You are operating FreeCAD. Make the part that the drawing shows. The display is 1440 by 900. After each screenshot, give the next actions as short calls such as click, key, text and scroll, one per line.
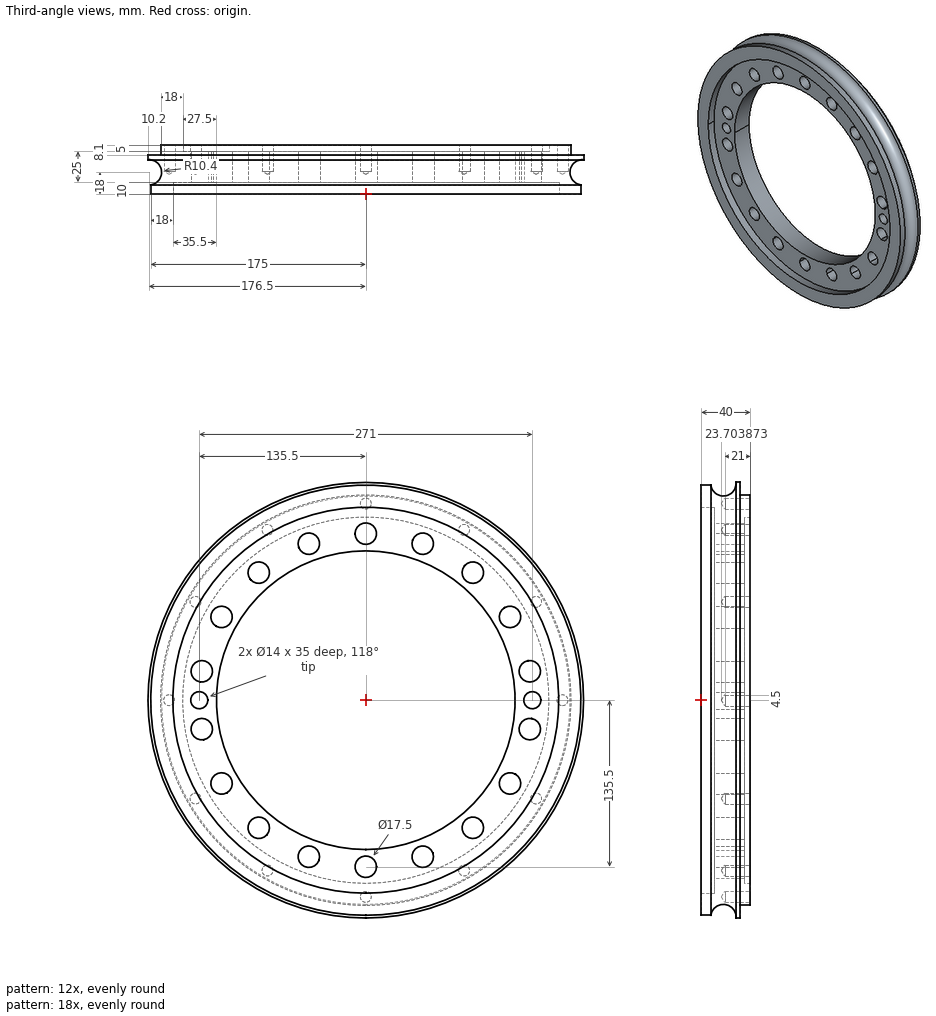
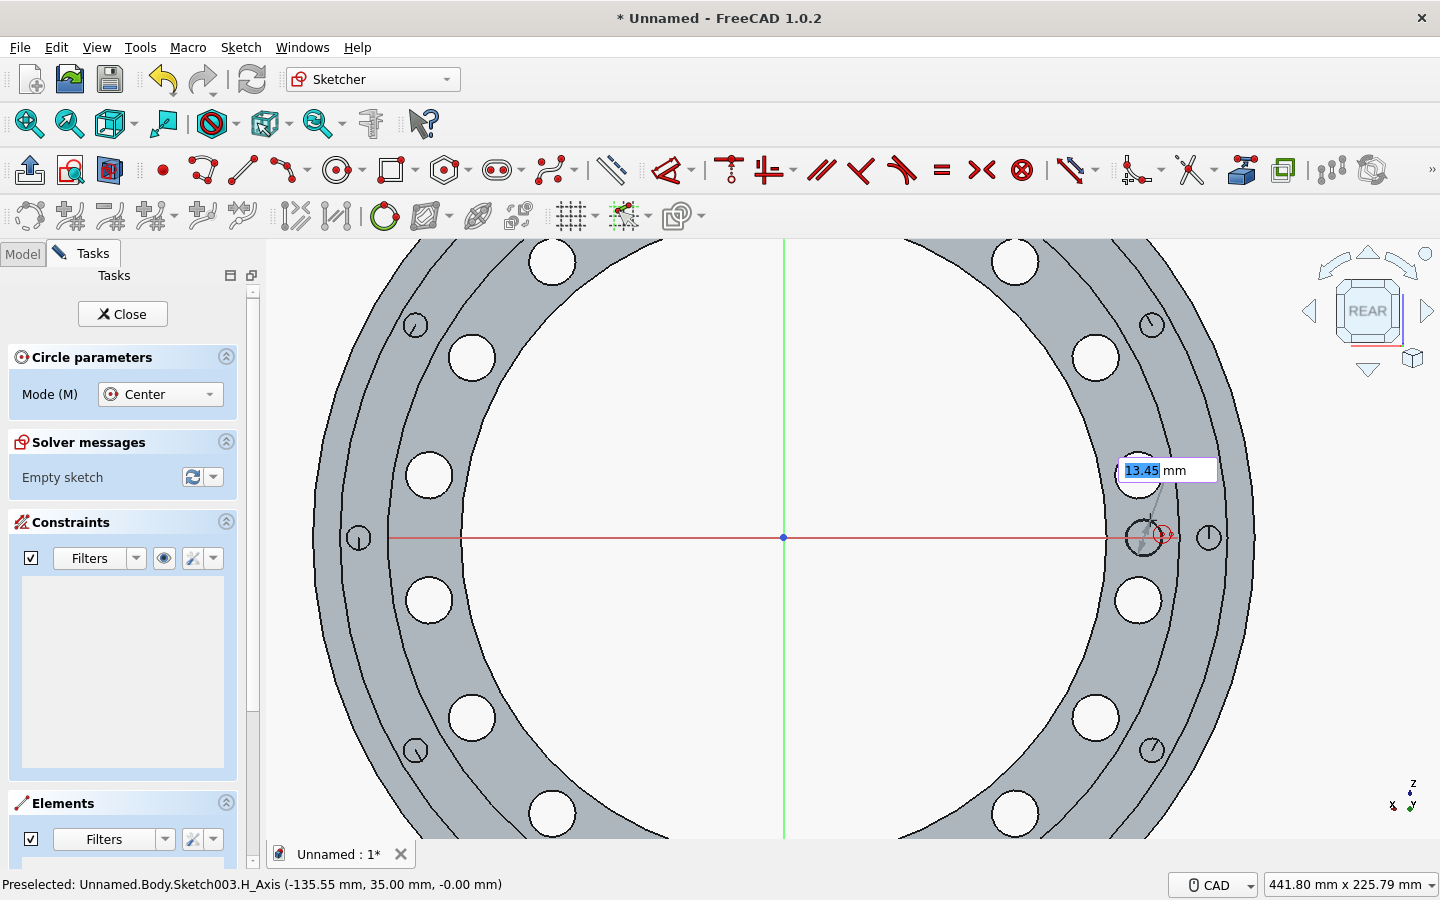
text(14)
key(Return)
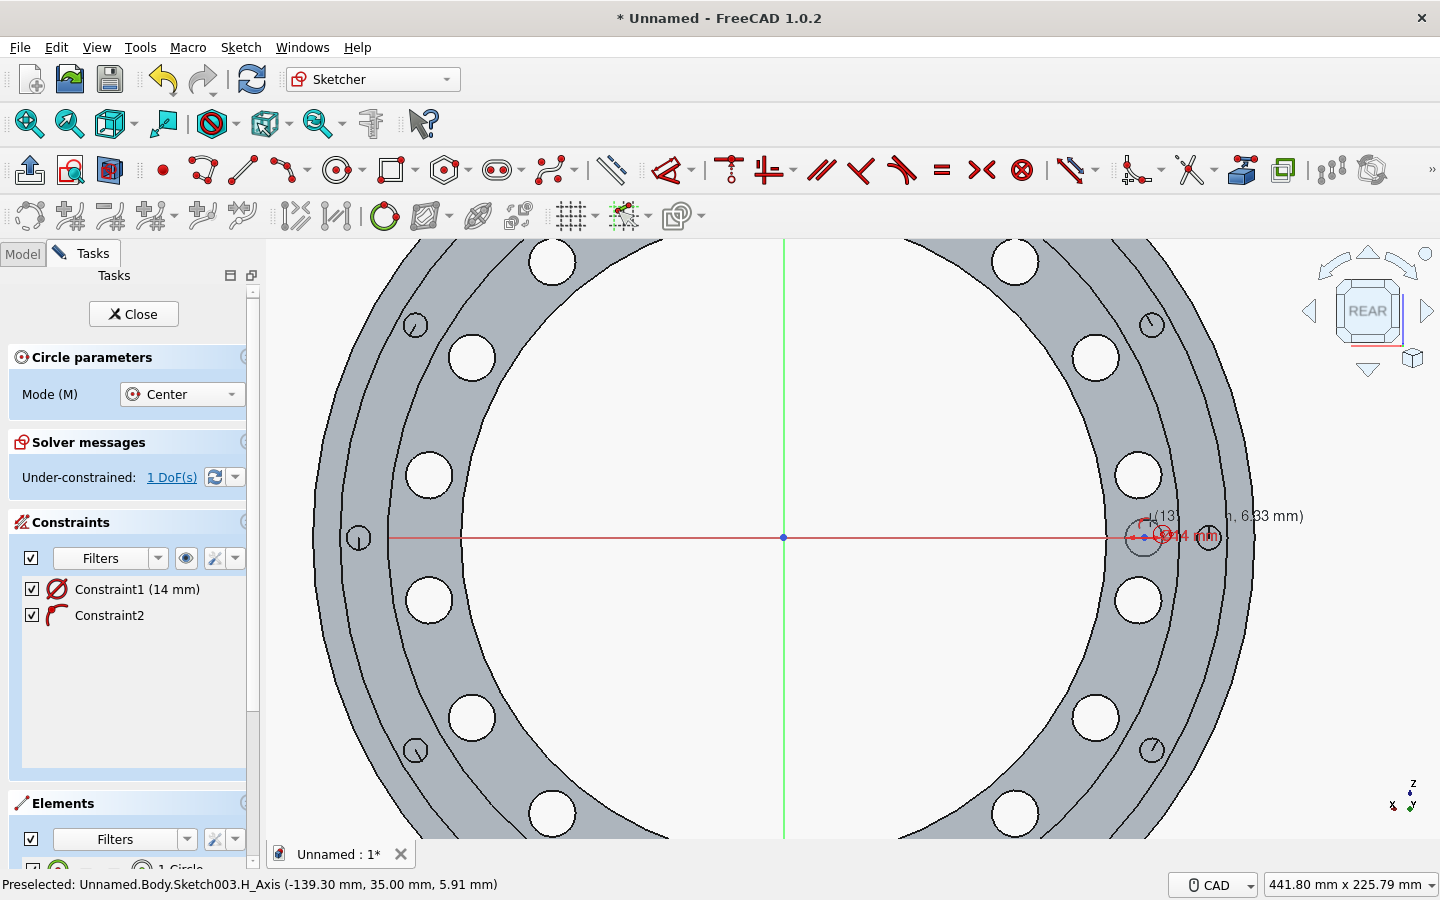
click(424, 538)
move(430, 520)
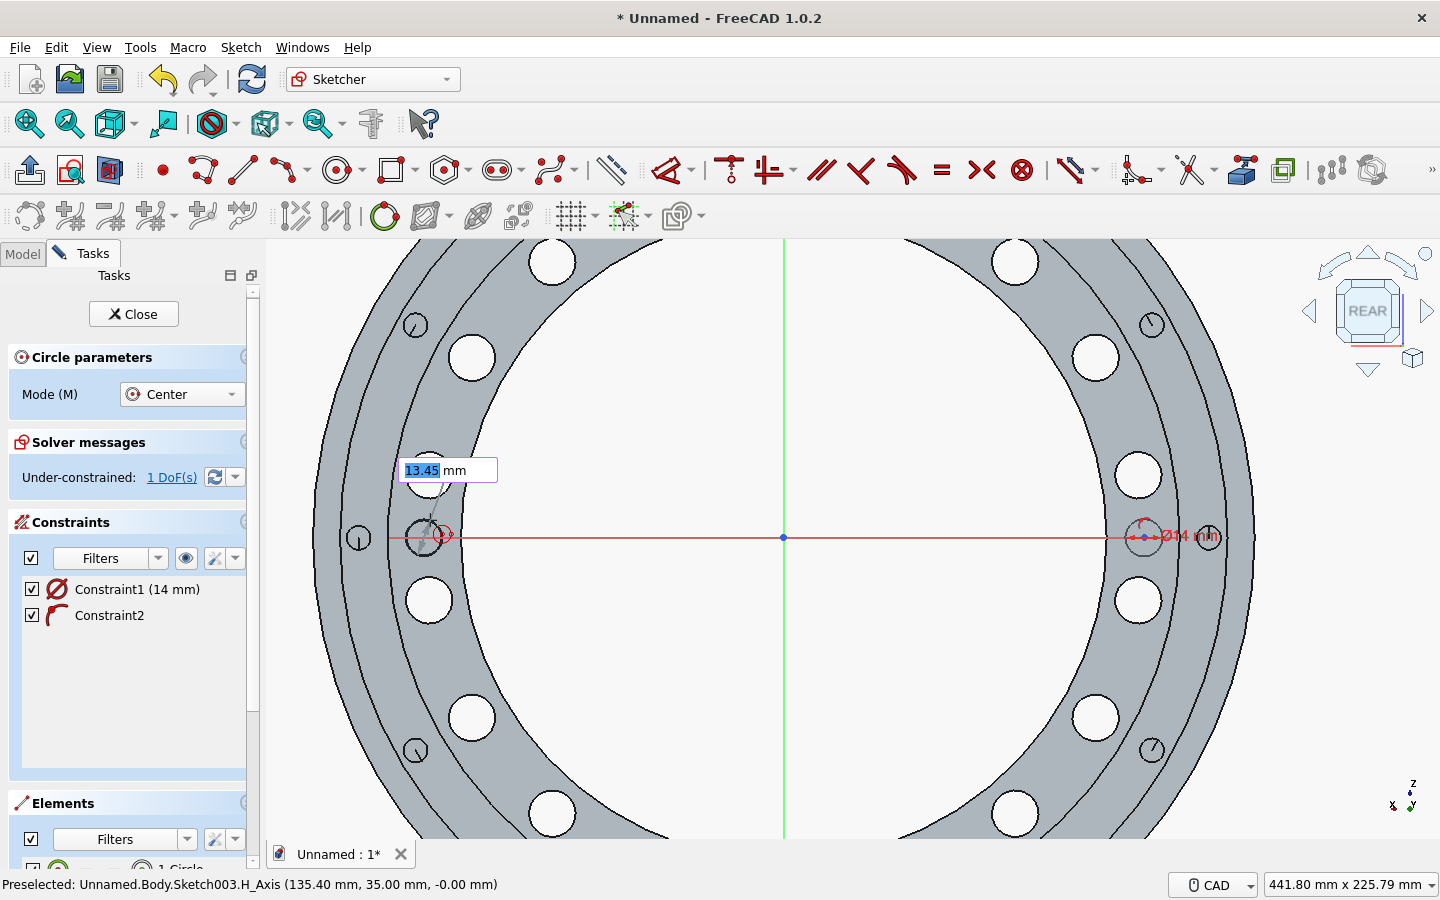
text(14)
key(Return)
key(Escape)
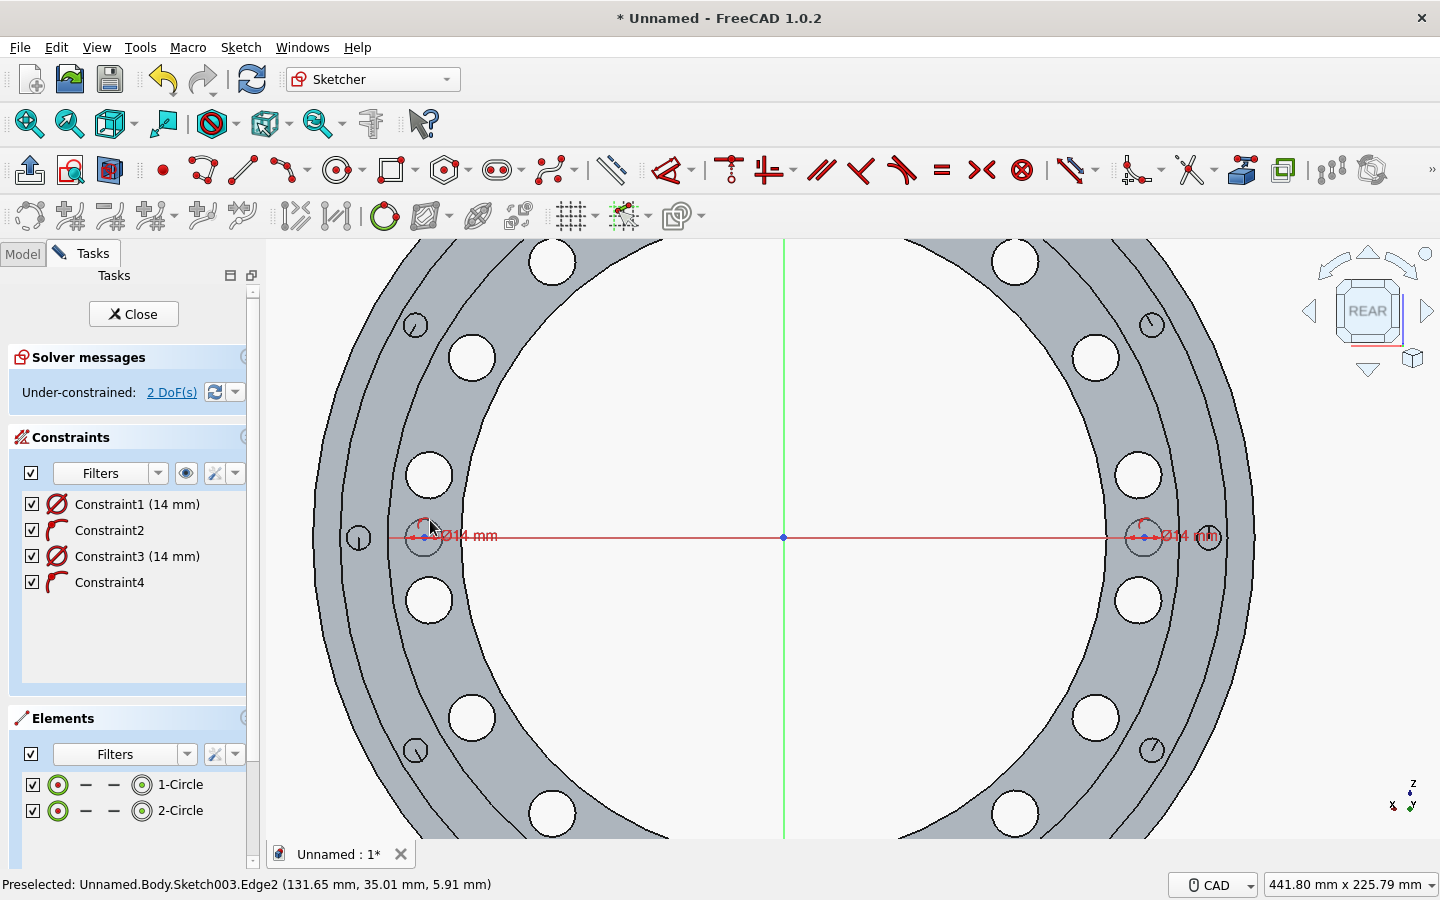
click(666, 170)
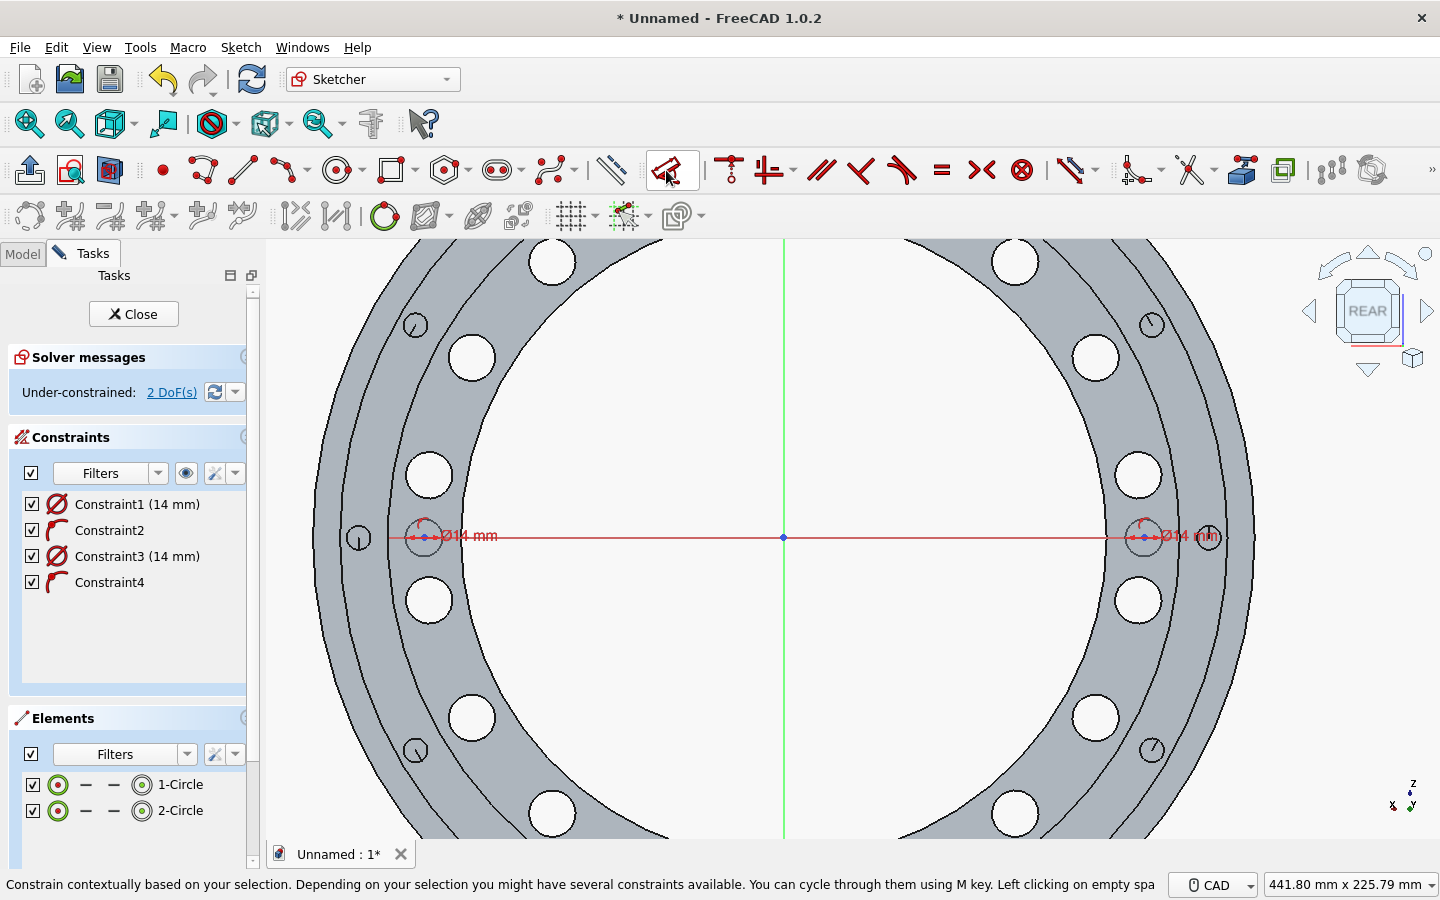
click(1144, 538)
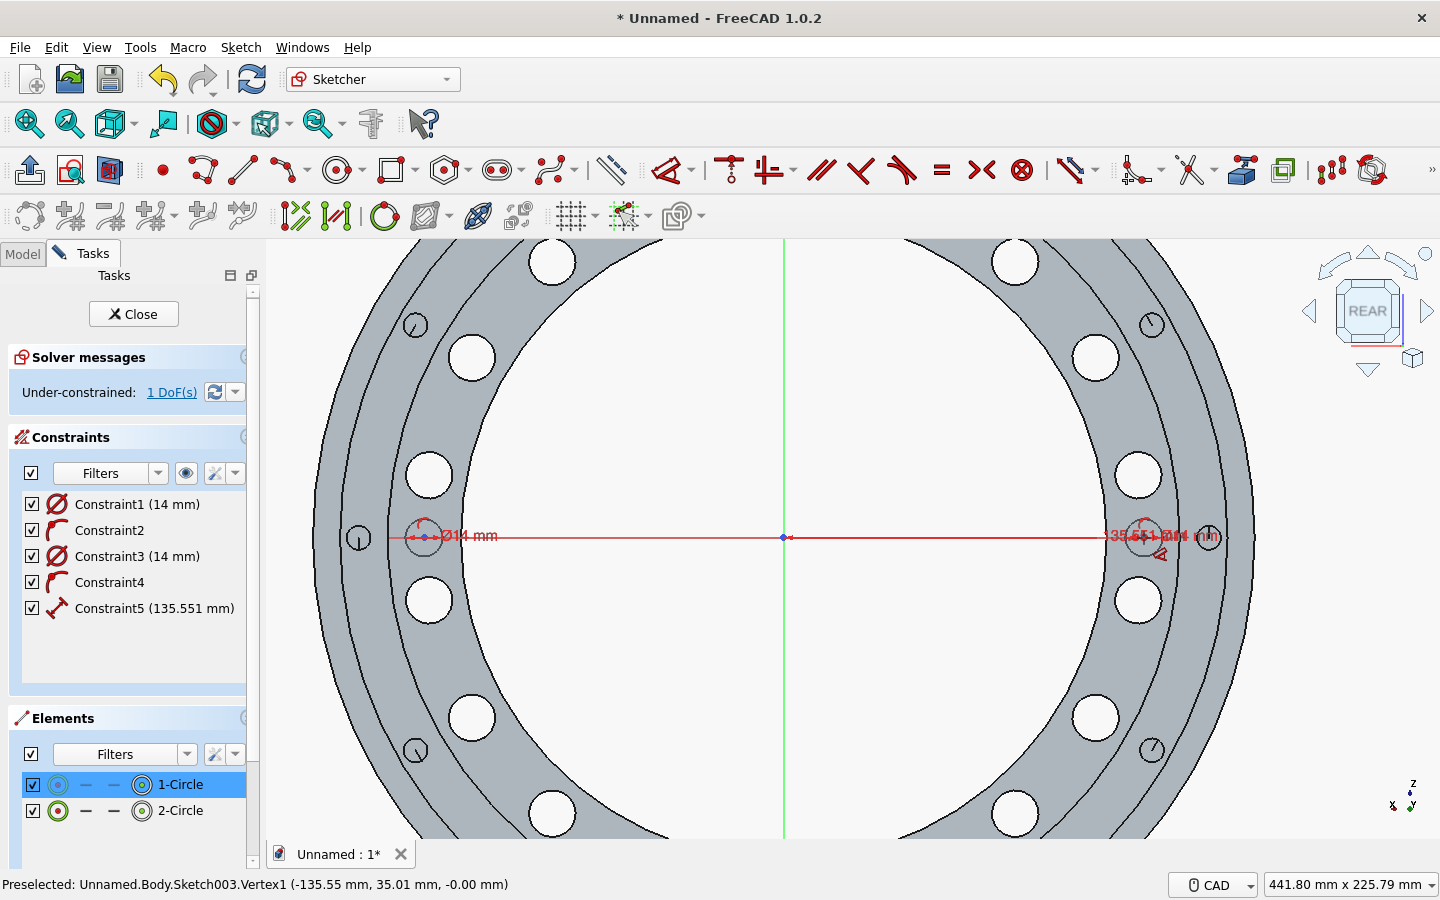
click(424, 538)
click(618, 572)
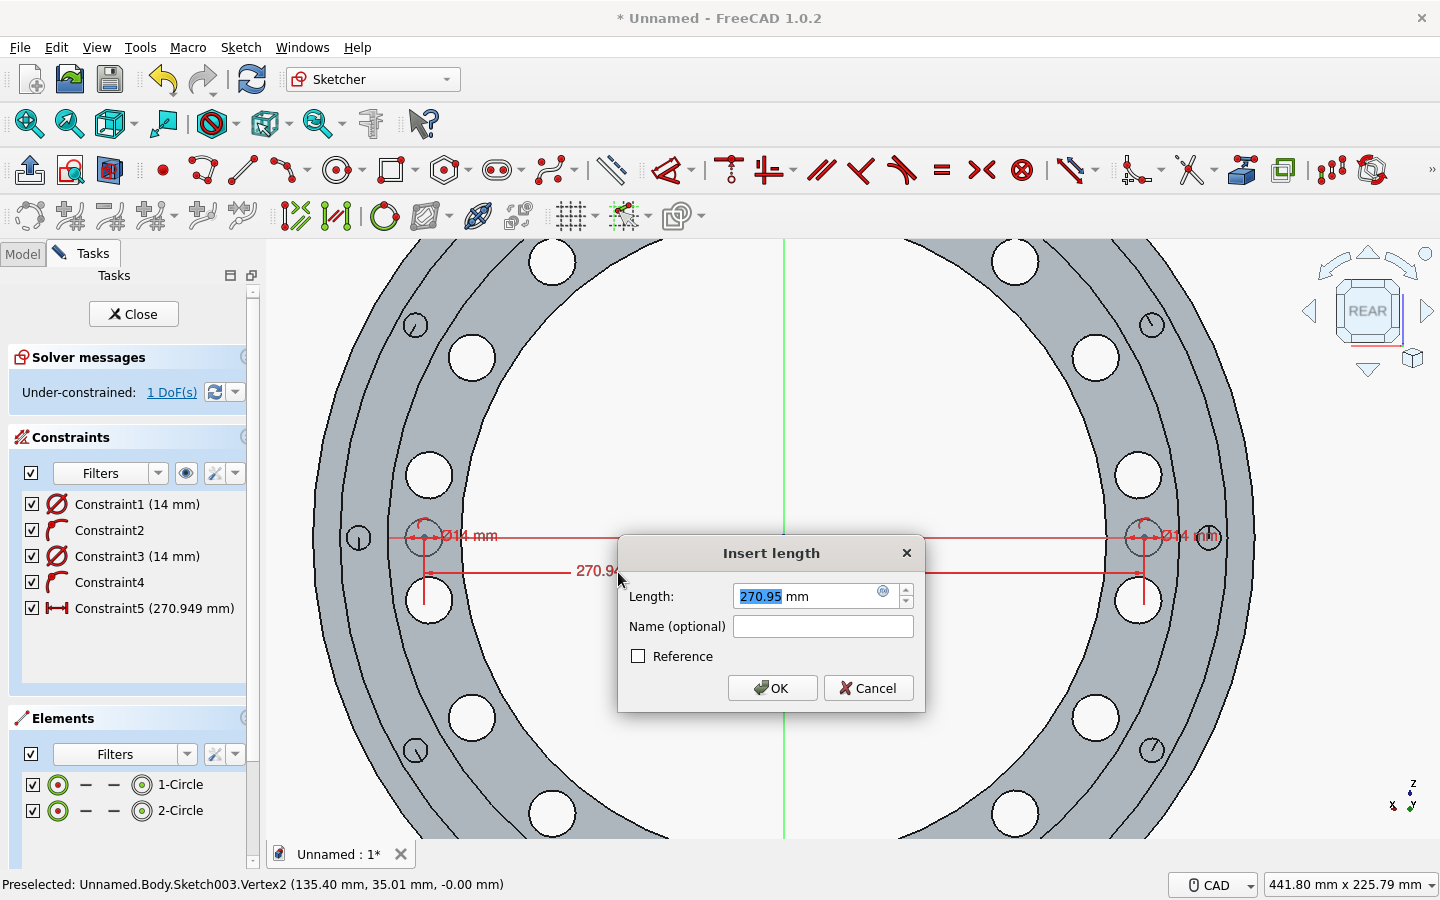
text(271)
key(Return)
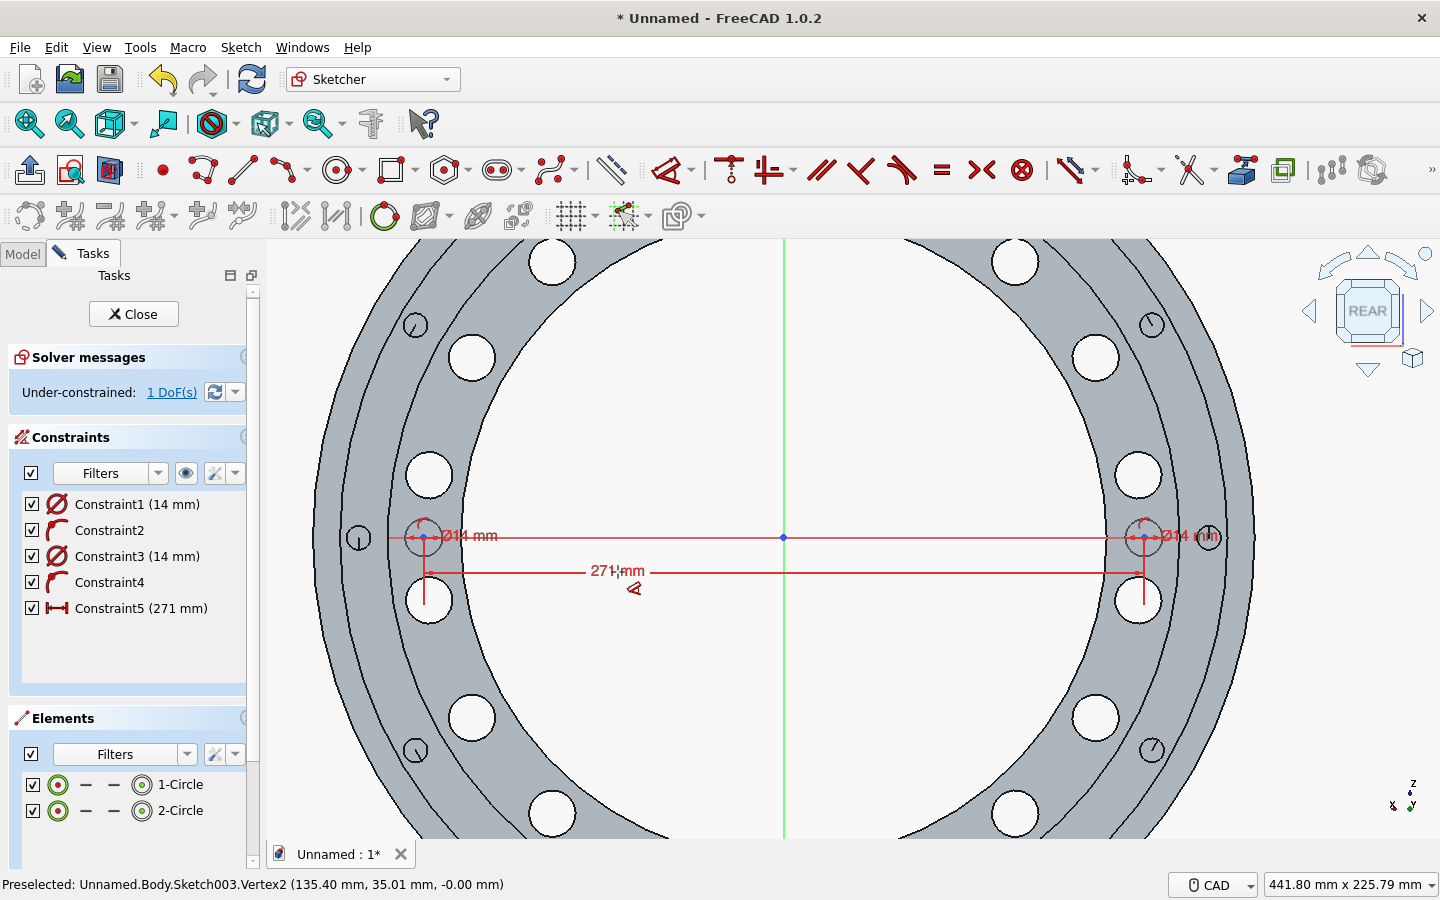
click(1144, 538)
click(964, 572)